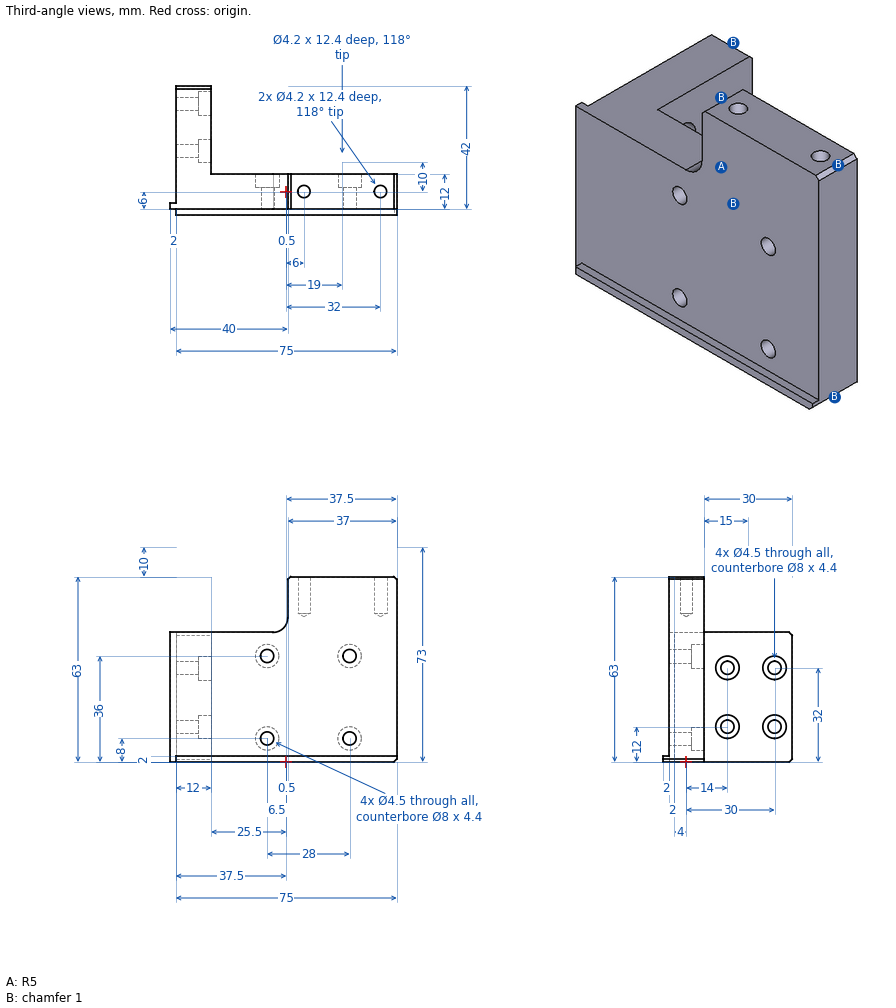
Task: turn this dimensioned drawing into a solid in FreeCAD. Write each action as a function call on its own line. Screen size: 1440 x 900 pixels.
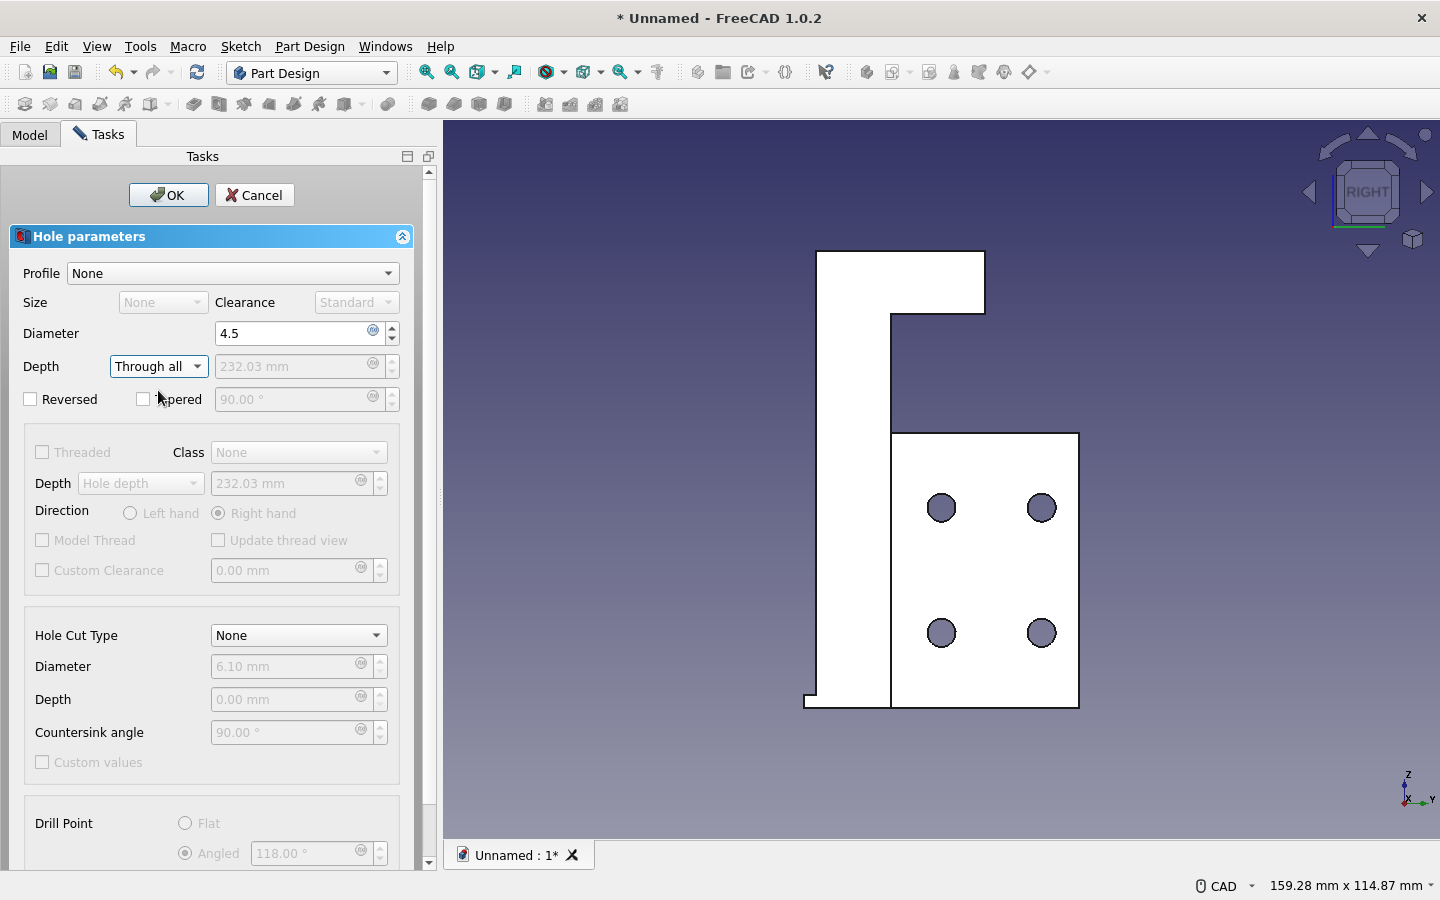
click(300, 636)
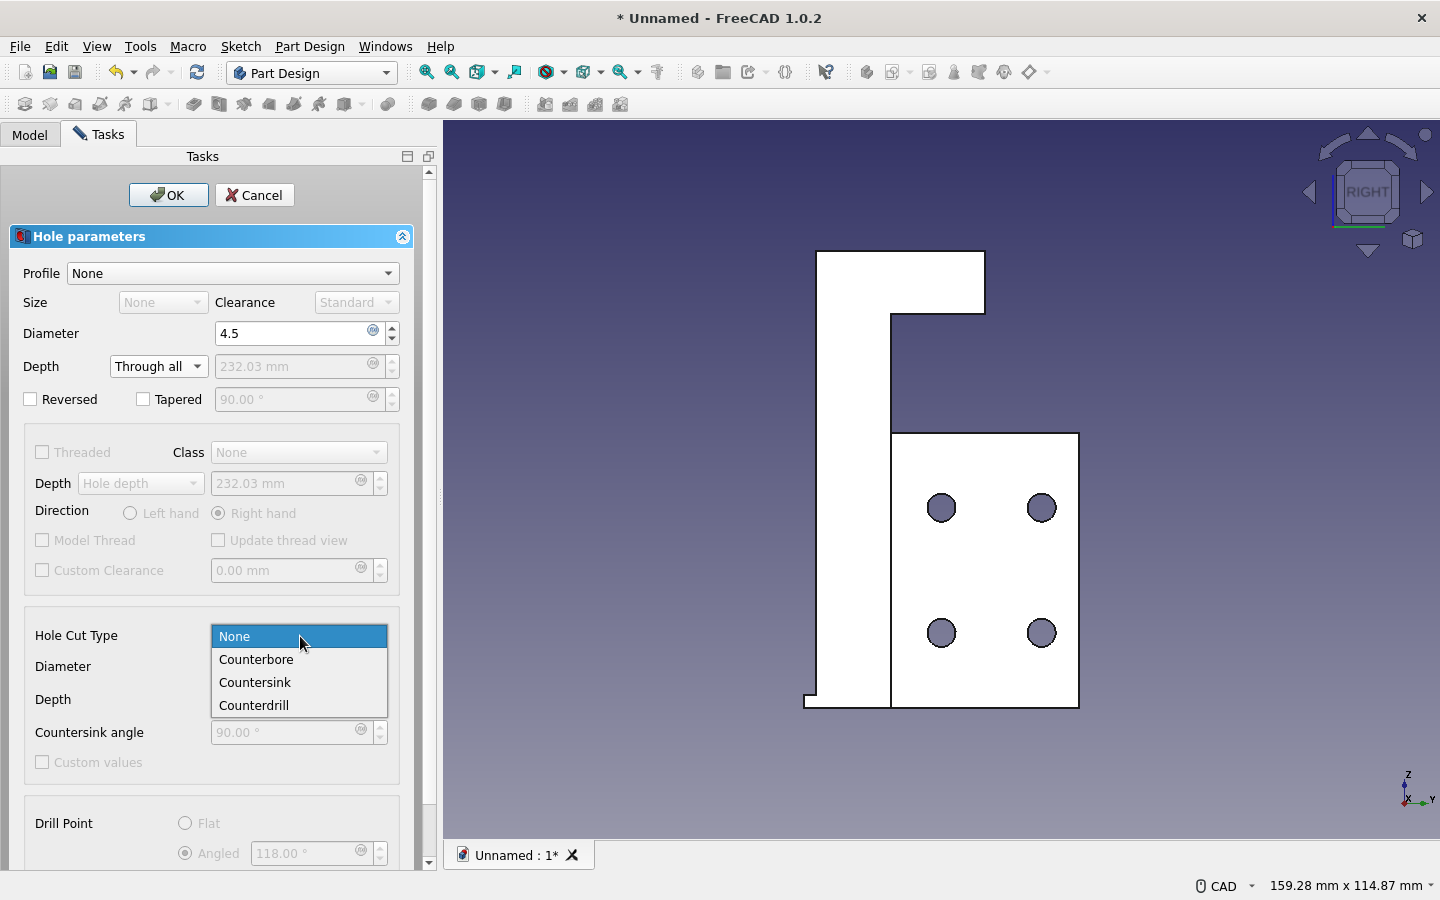
click(298, 660)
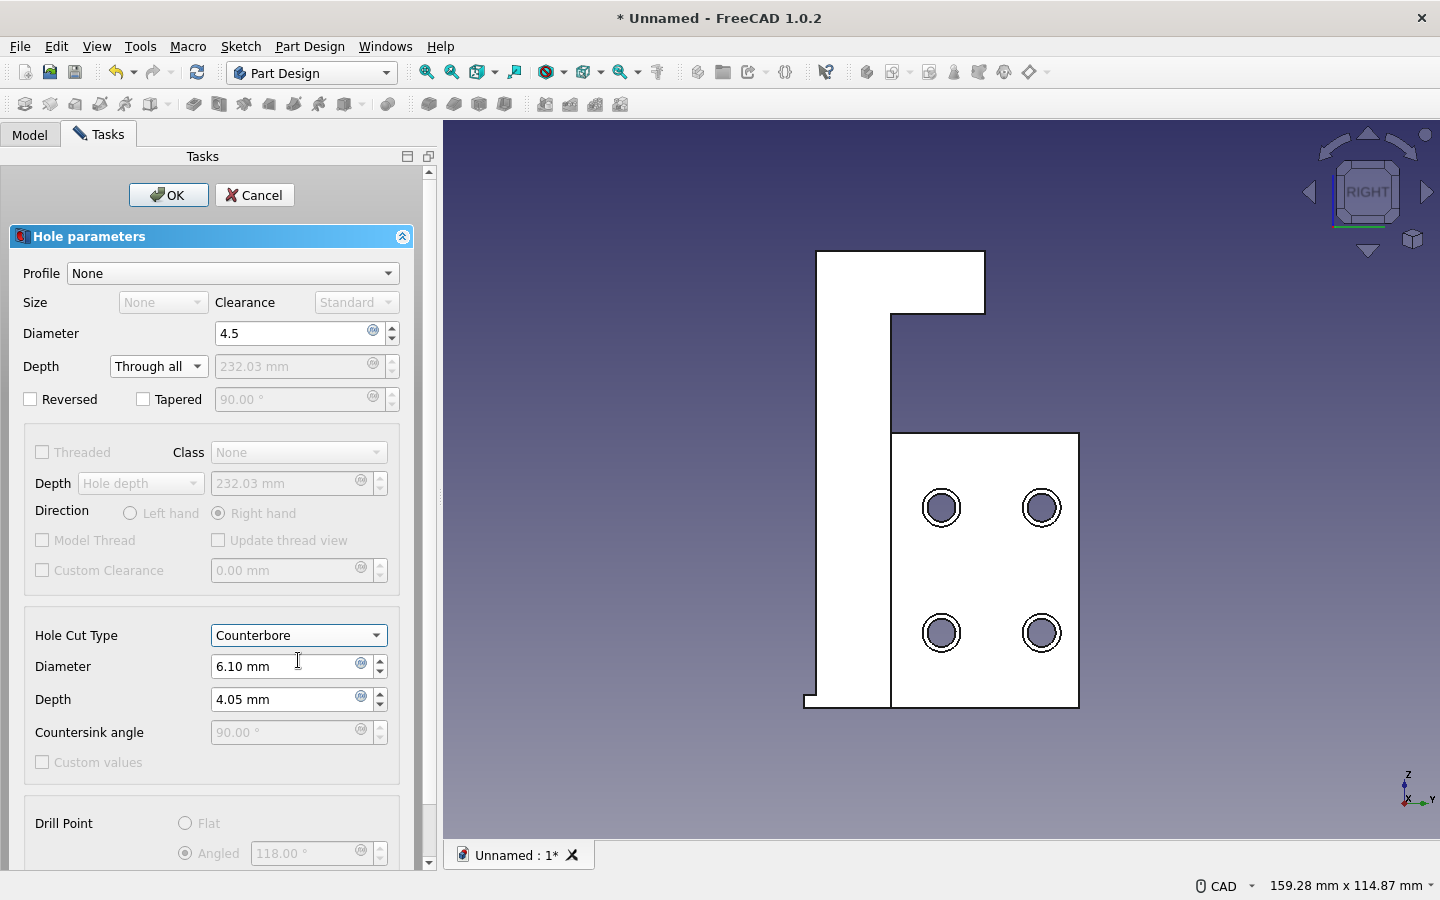
triple_click(292, 666)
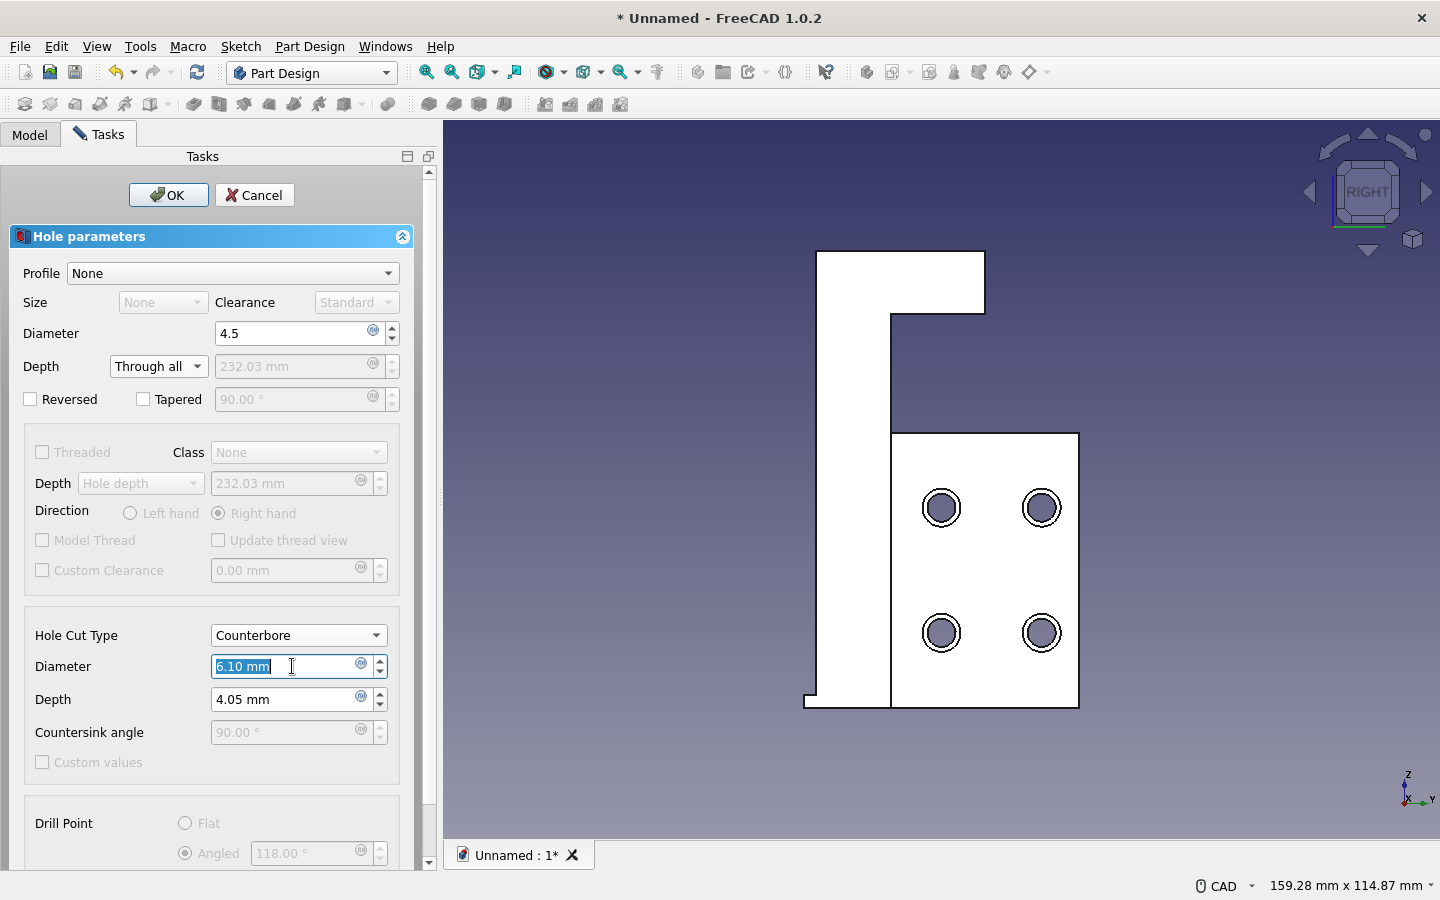
text(8)
key(Tab)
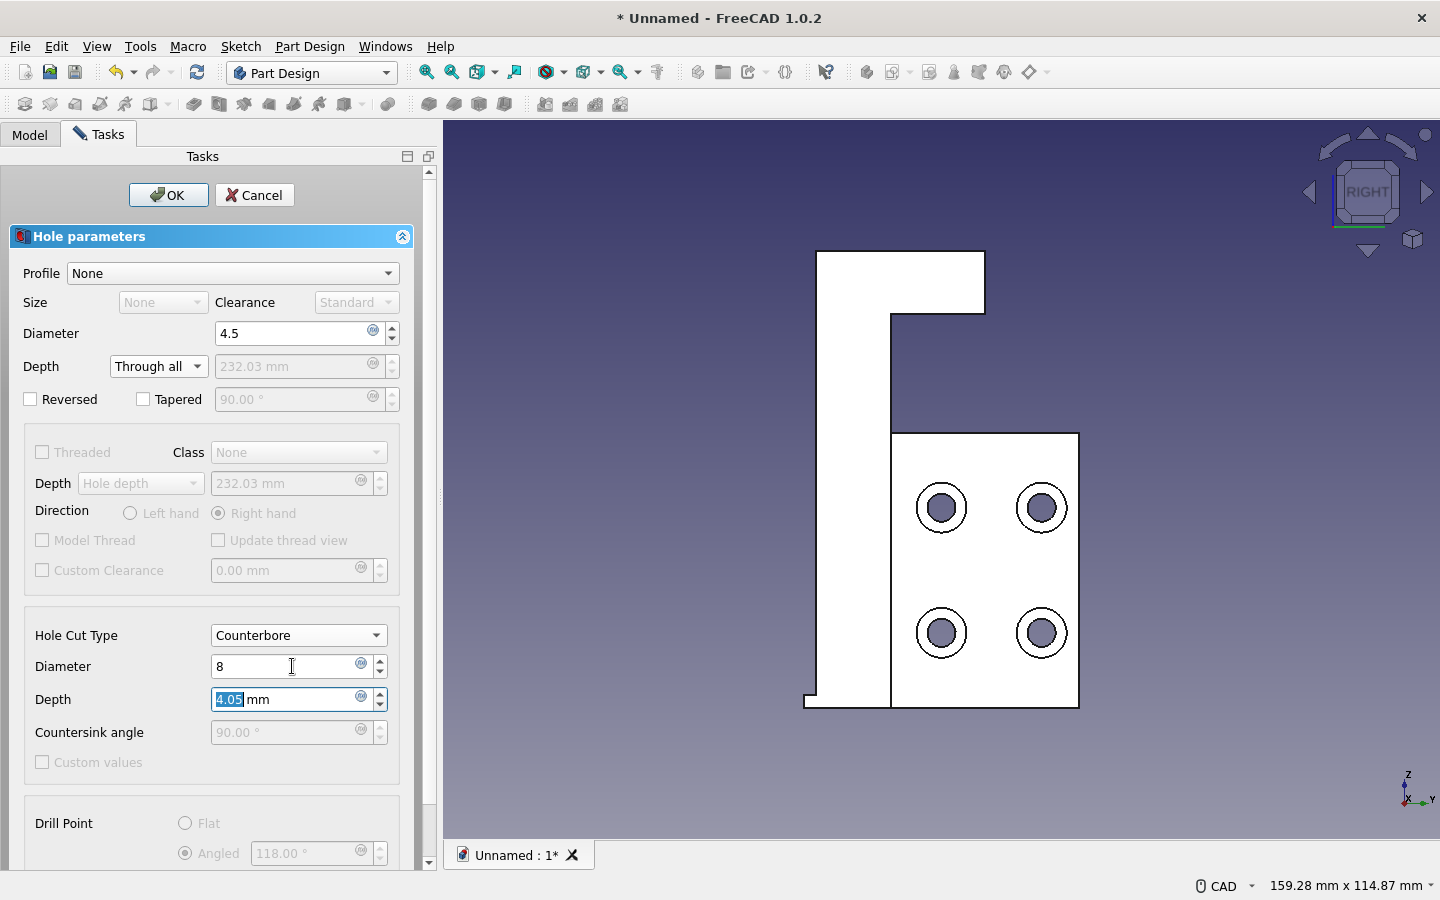
text(4.4)
key(Tab)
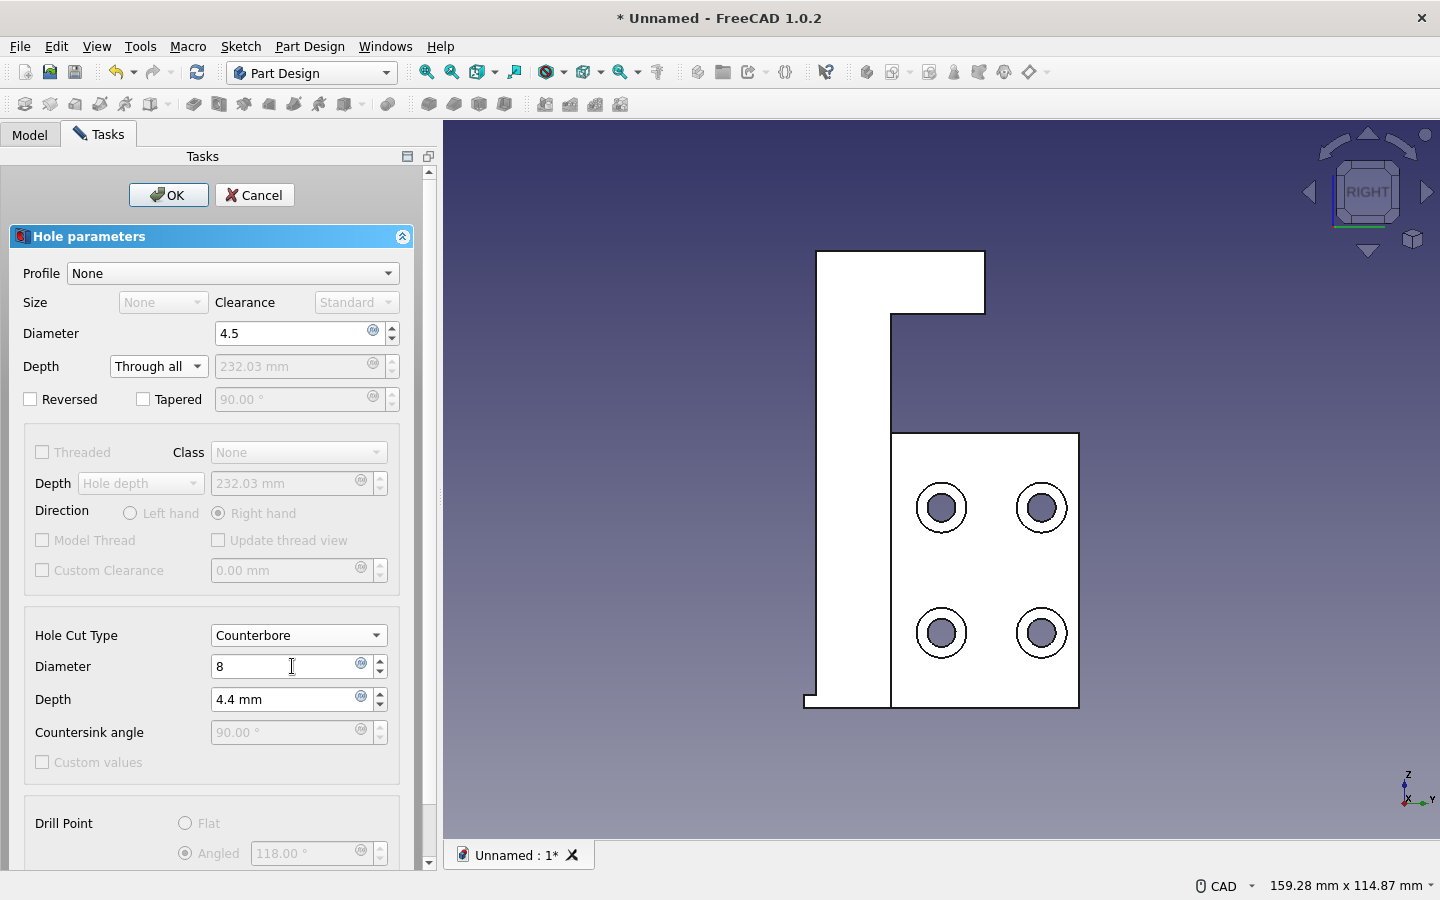
click(169, 195)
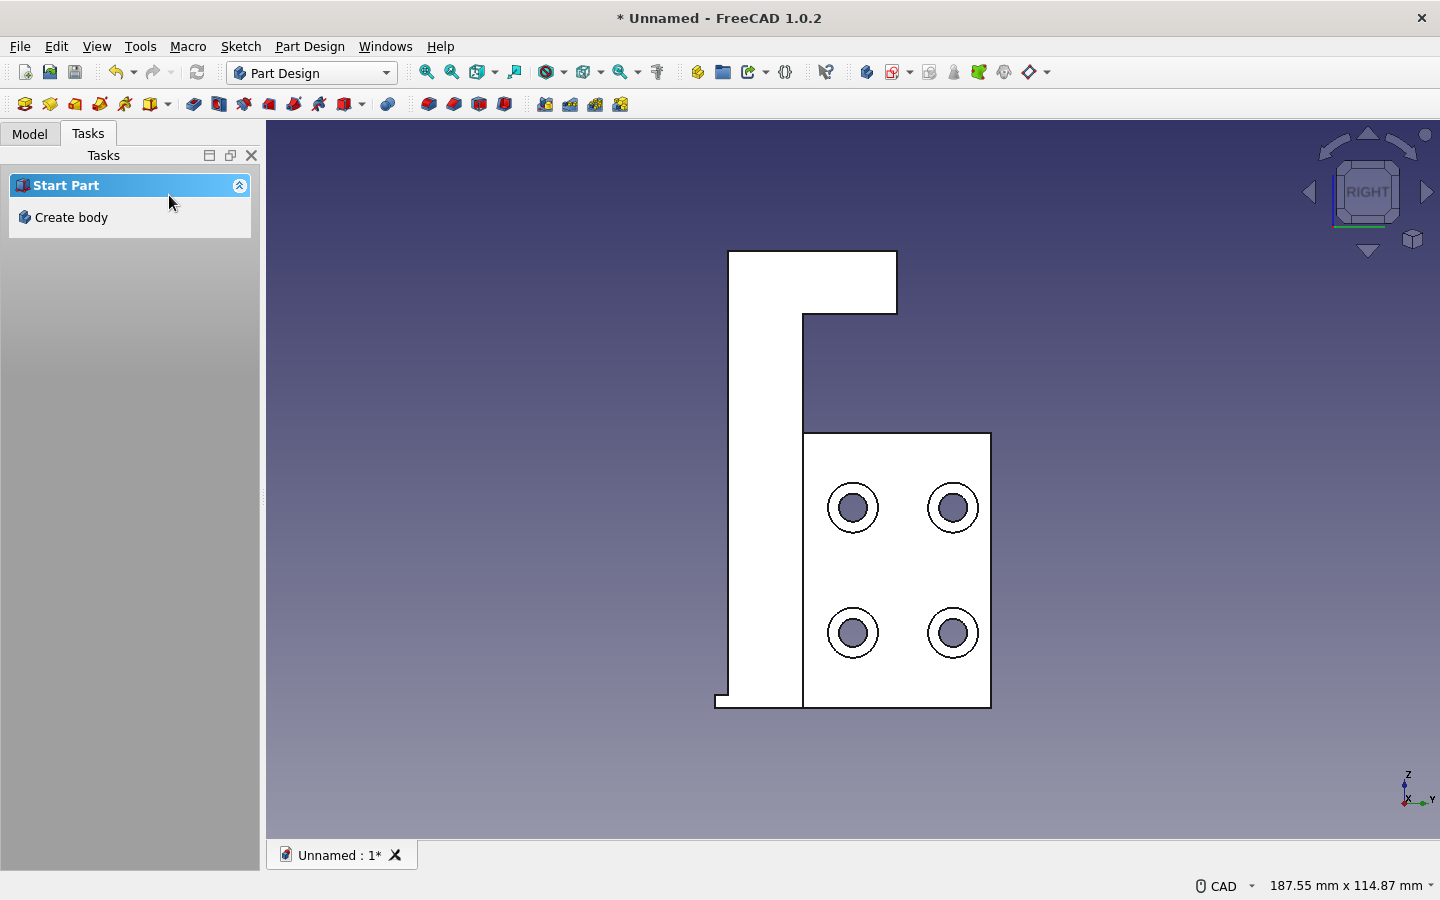
key(4)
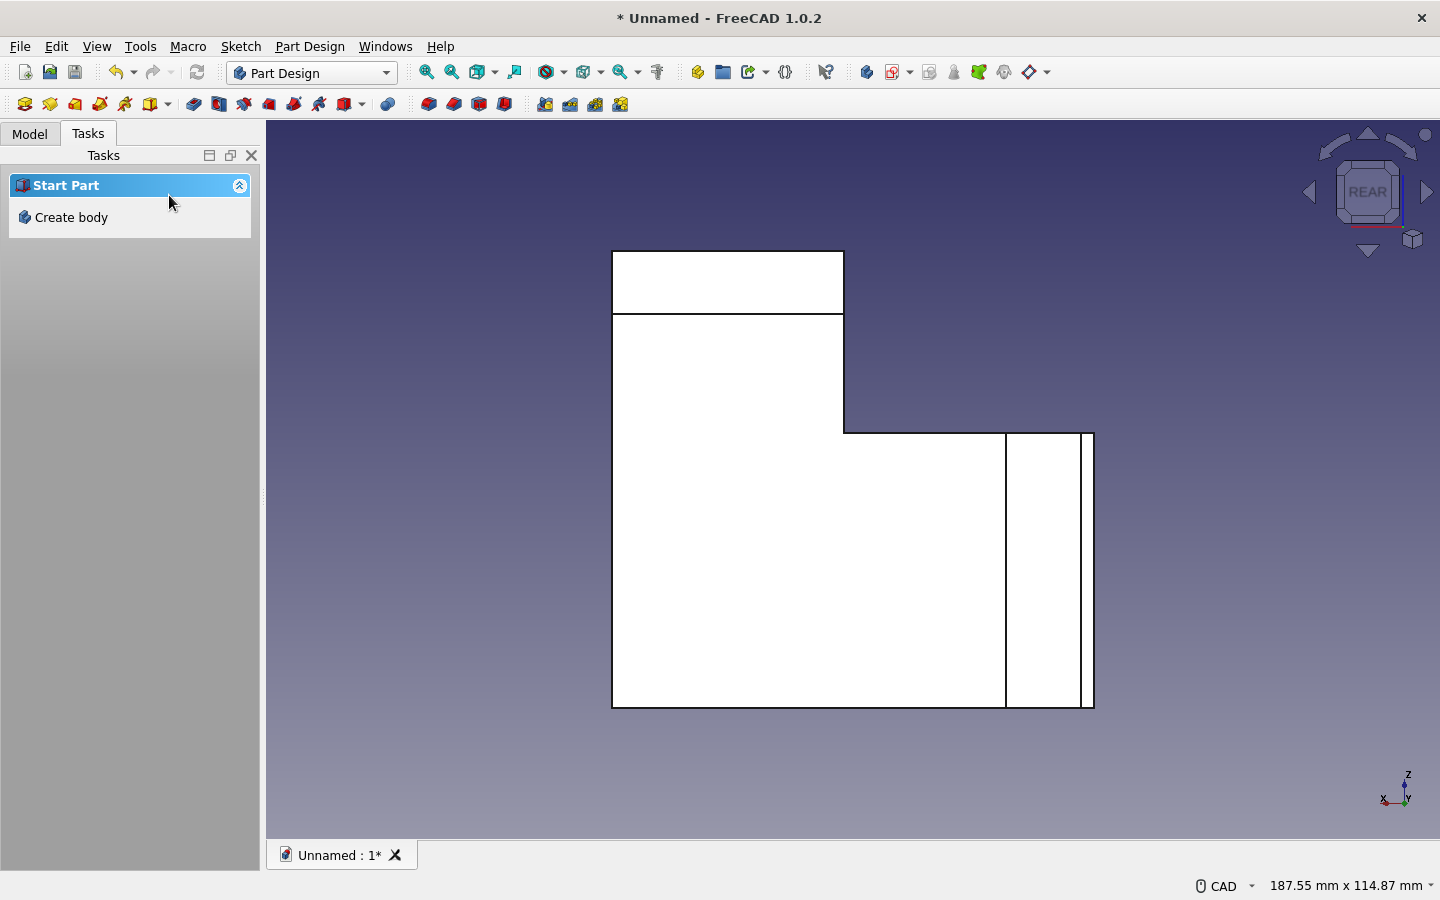
click(662, 281)